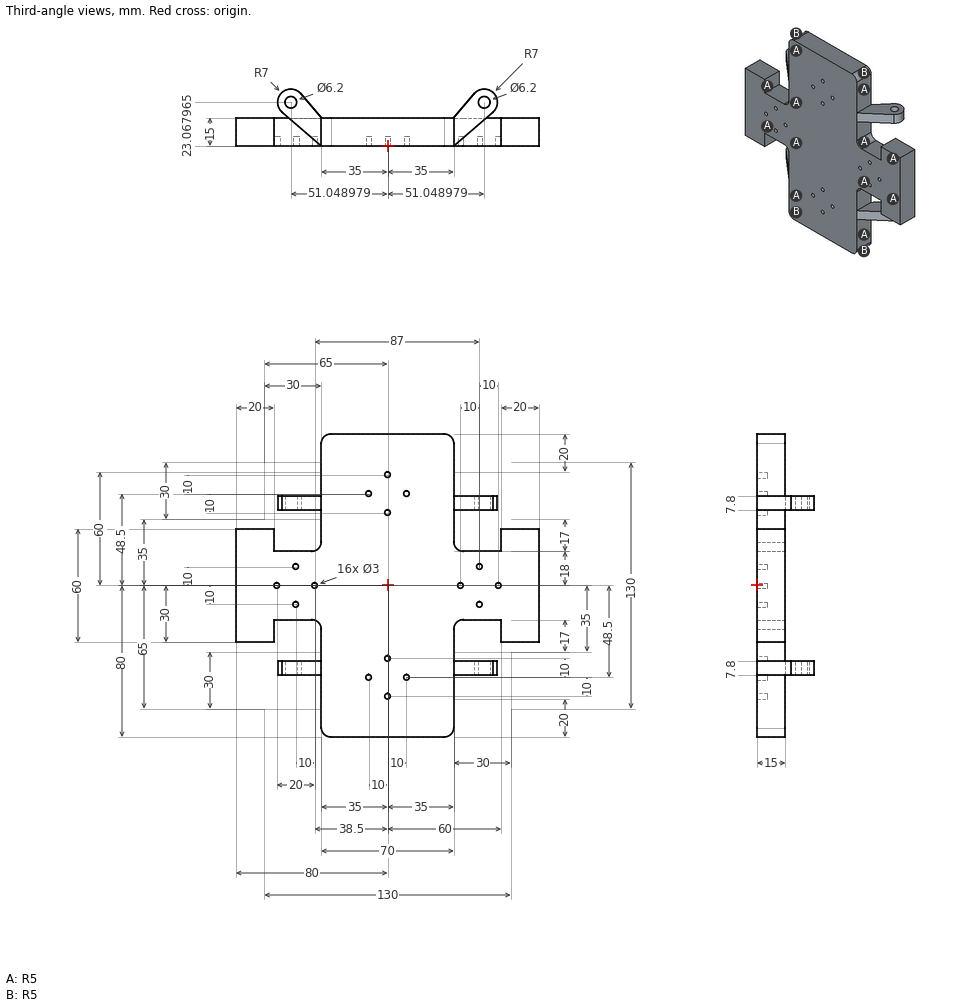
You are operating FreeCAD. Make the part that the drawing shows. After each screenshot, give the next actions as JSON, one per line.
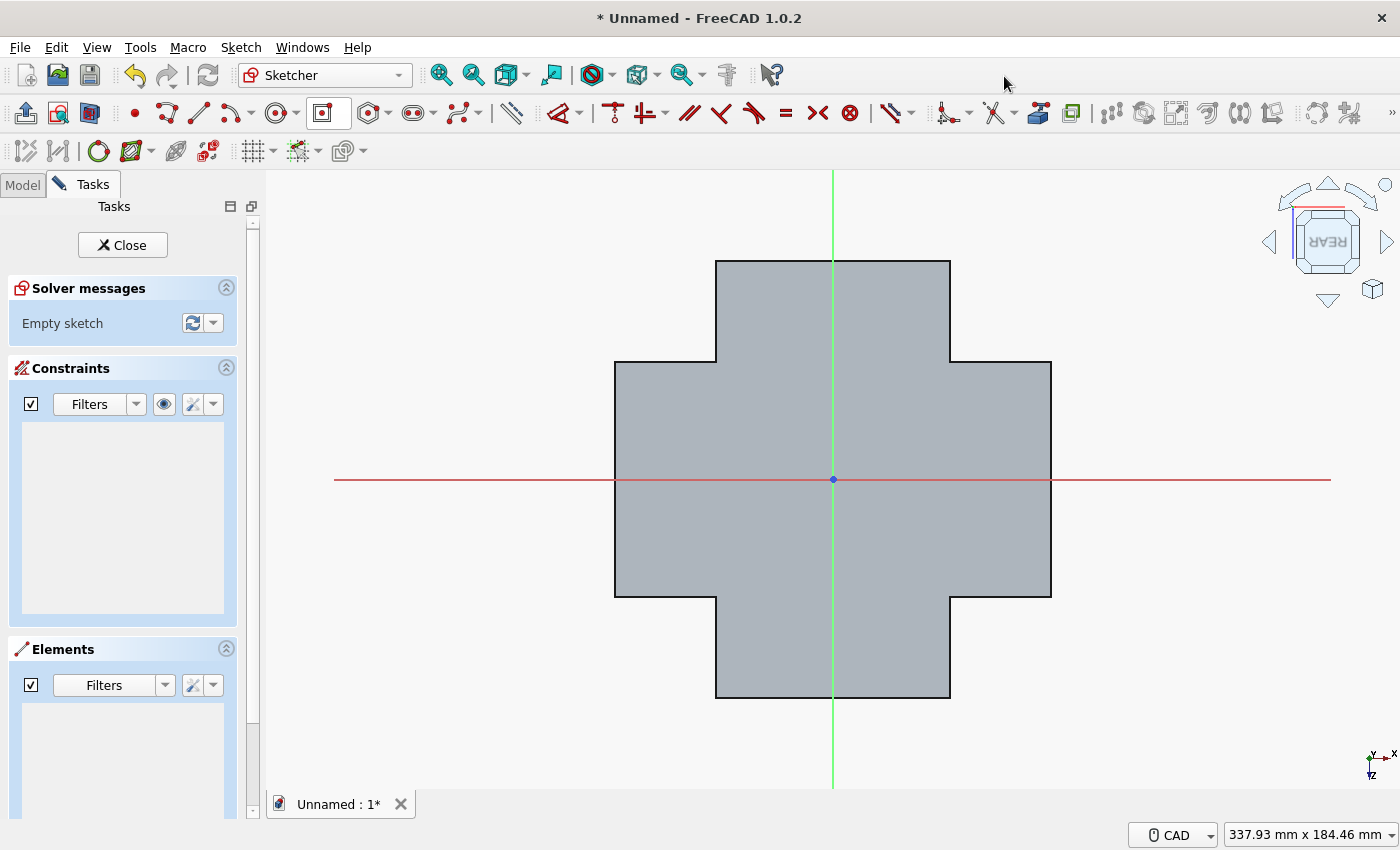
{"action": "scroll", "coordinate": [972, 479], "scroll_direction": "up", "scroll_amount": 2}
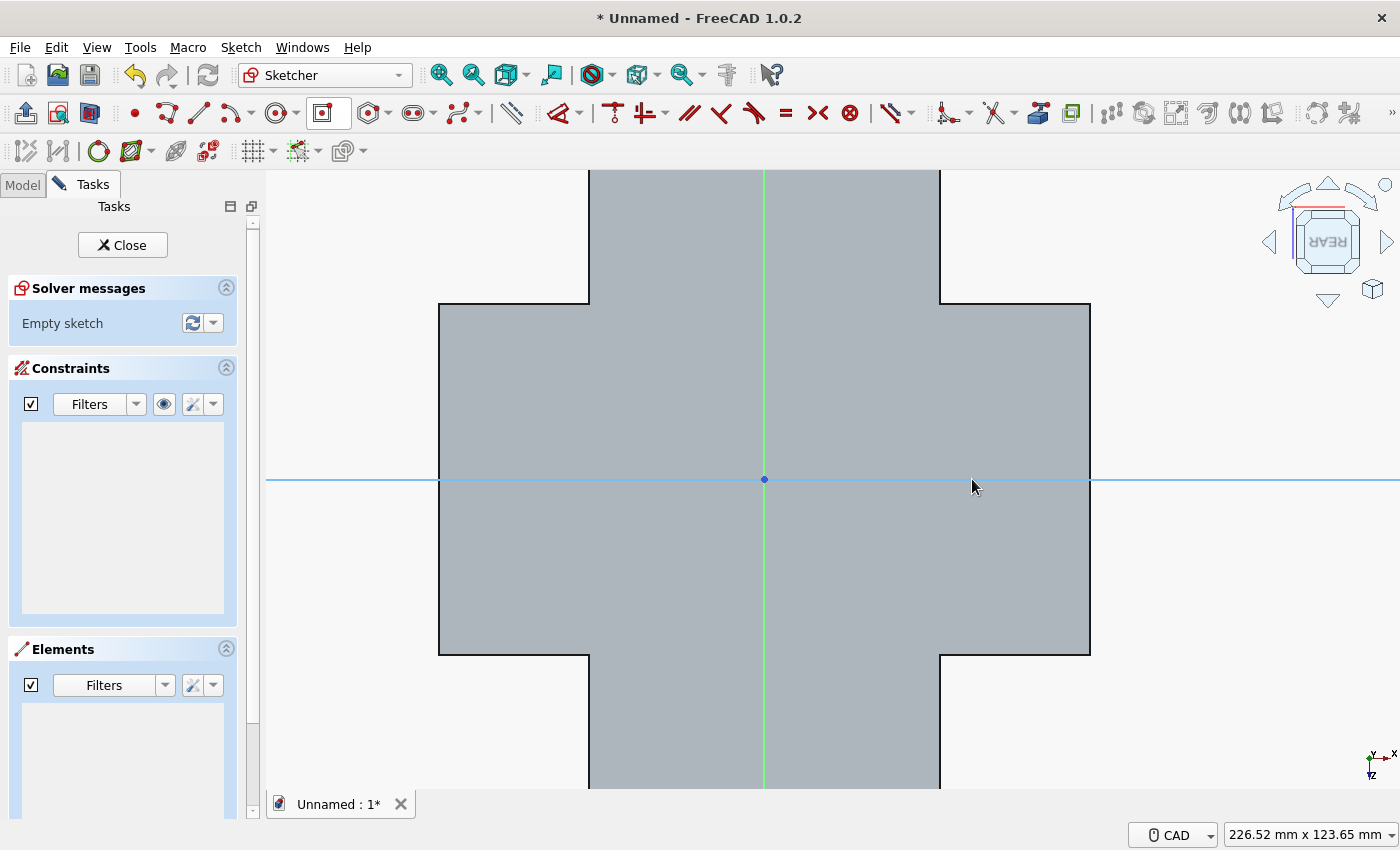
{"action": "key", "text": "g r"}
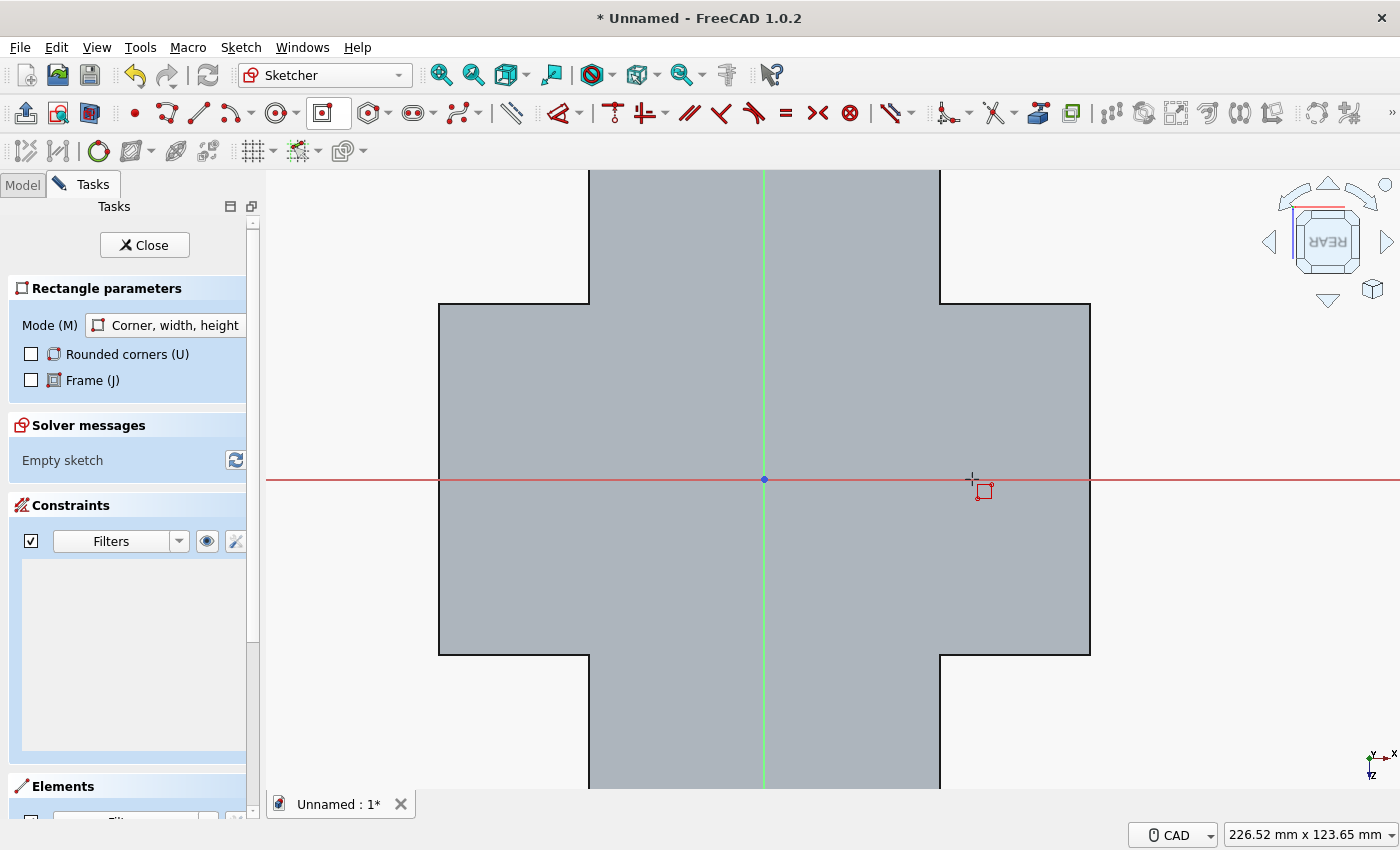
{"action": "left_click", "coordinate": [940, 304]}
{"action": "mouse_move", "coordinate": [1090, 389]}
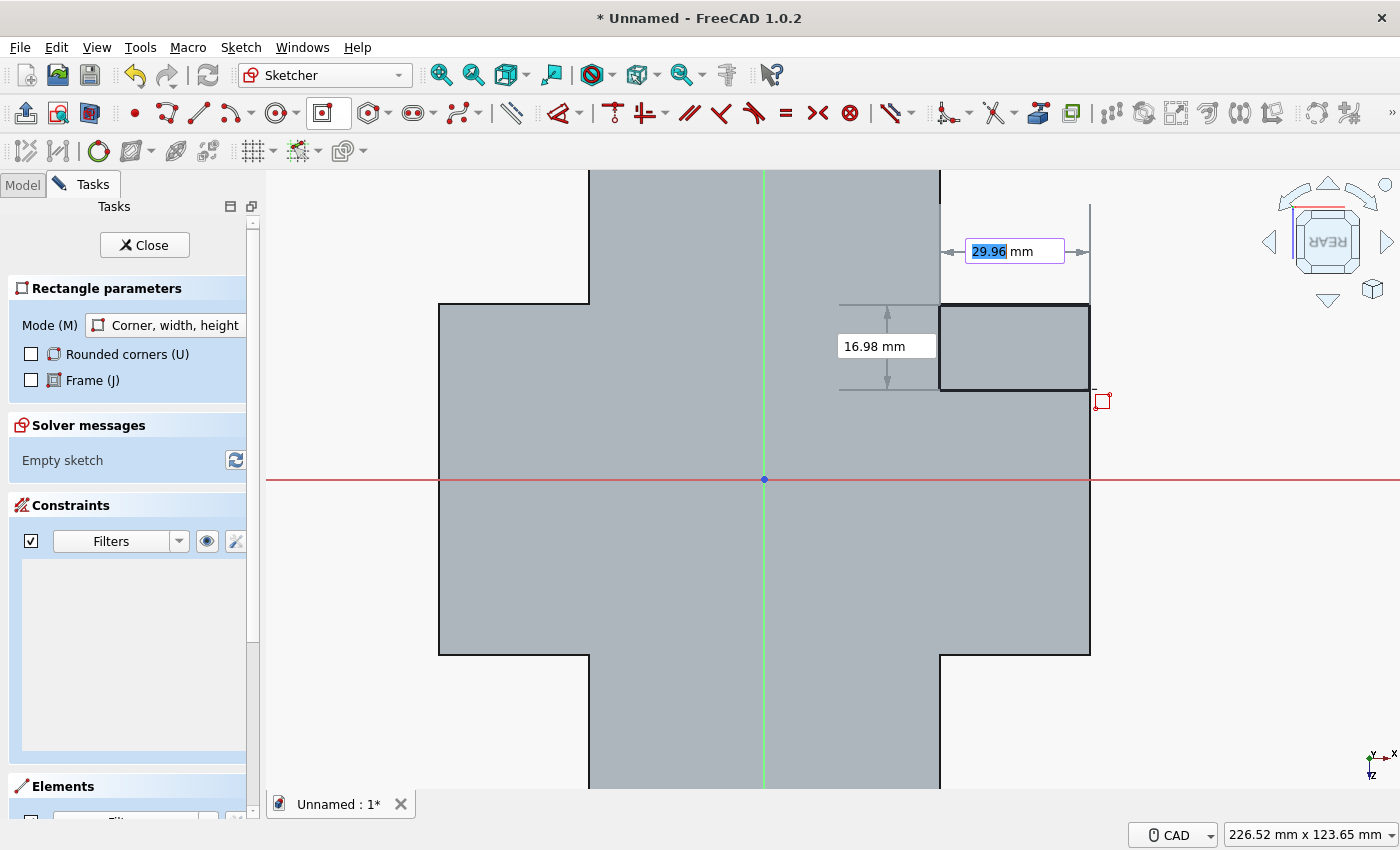
{"action": "type", "text": "30"}
{"action": "key", "text": "Tab"}
{"action": "type", "text": "17"}
{"action": "key", "text": "Return"}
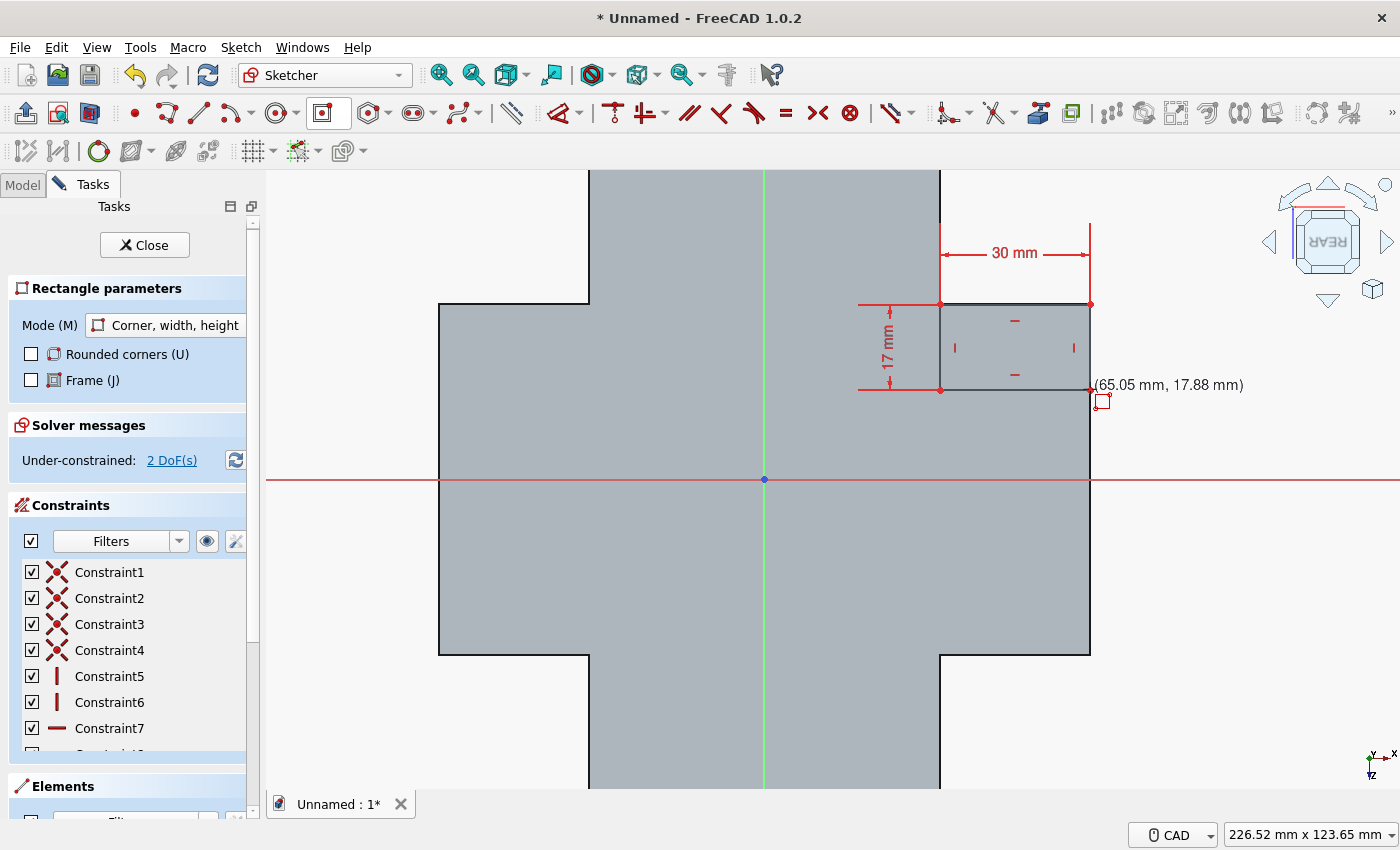
{"action": "left_click", "coordinate": [940, 570]}
{"action": "mouse_move", "coordinate": [1090, 655]}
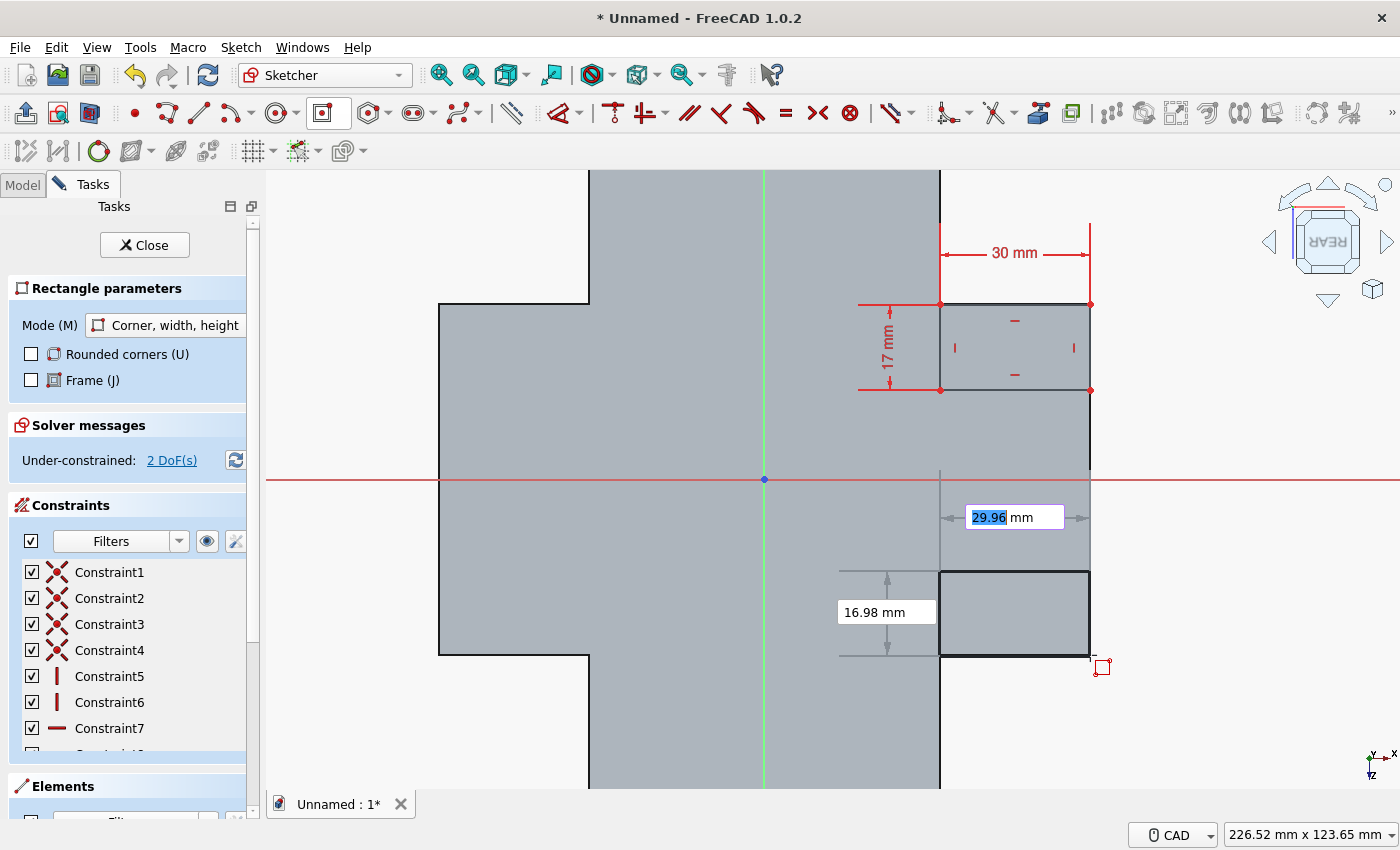
{"action": "type", "text": "30"}
{"action": "key", "text": "Tab"}
{"action": "type", "text": "17"}
{"action": "key", "text": "Return"}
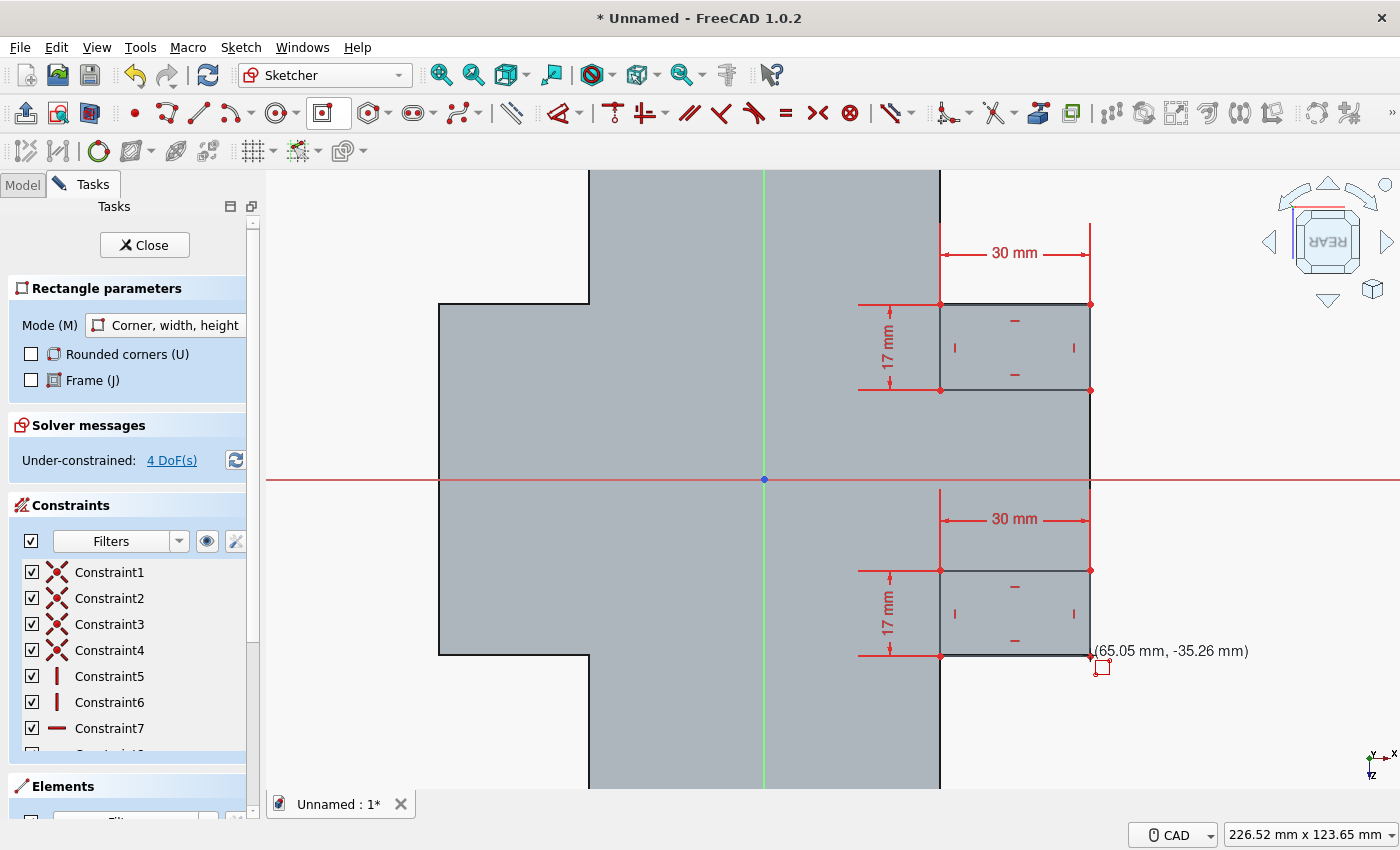
{"action": "left_click", "coordinate": [439, 304]}
{"action": "mouse_move", "coordinate": [589, 389]}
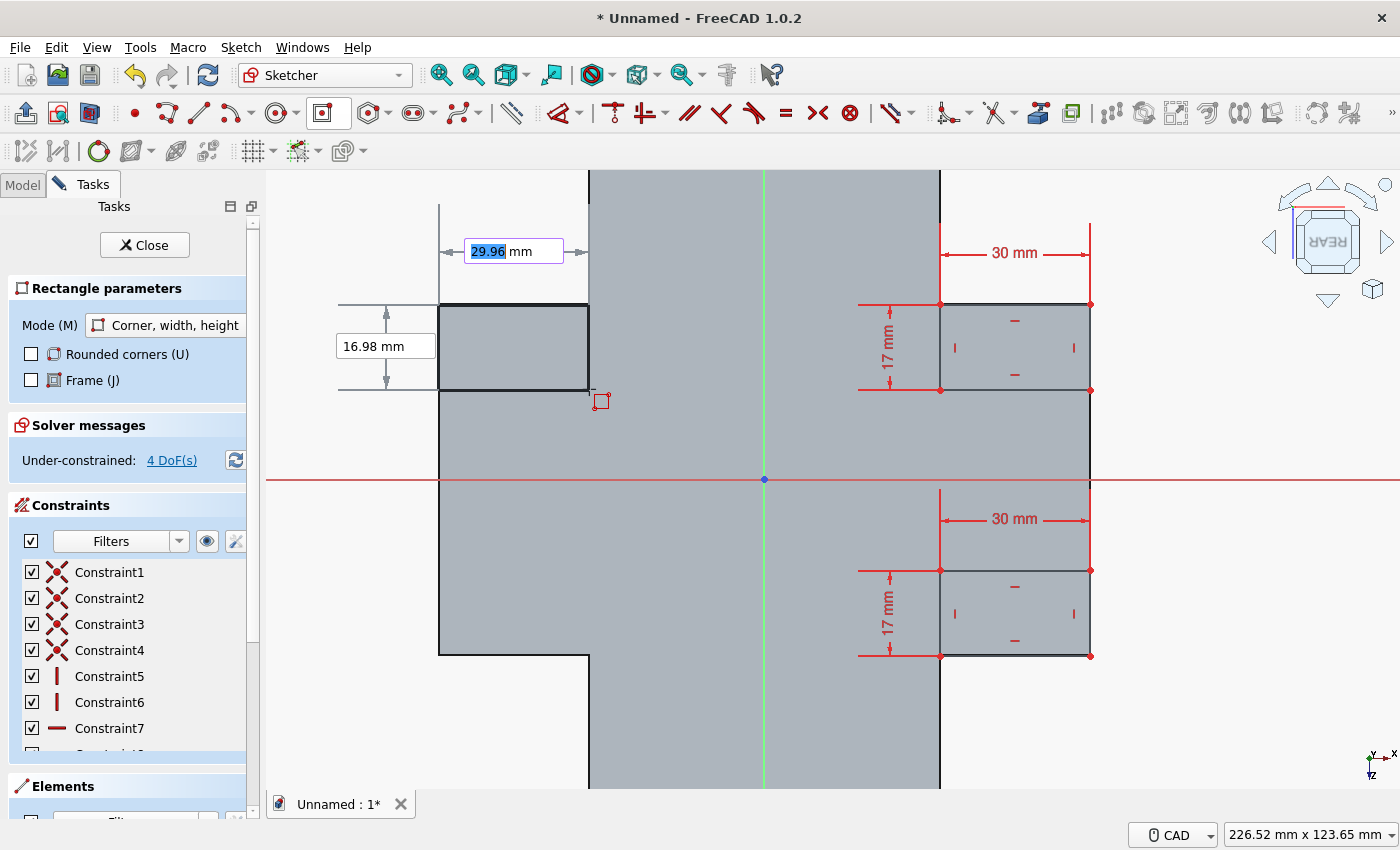
{"action": "type", "text": "30"}
{"action": "key", "text": "Tab"}
{"action": "type", "text": "17"}
{"action": "key", "text": "Return"}